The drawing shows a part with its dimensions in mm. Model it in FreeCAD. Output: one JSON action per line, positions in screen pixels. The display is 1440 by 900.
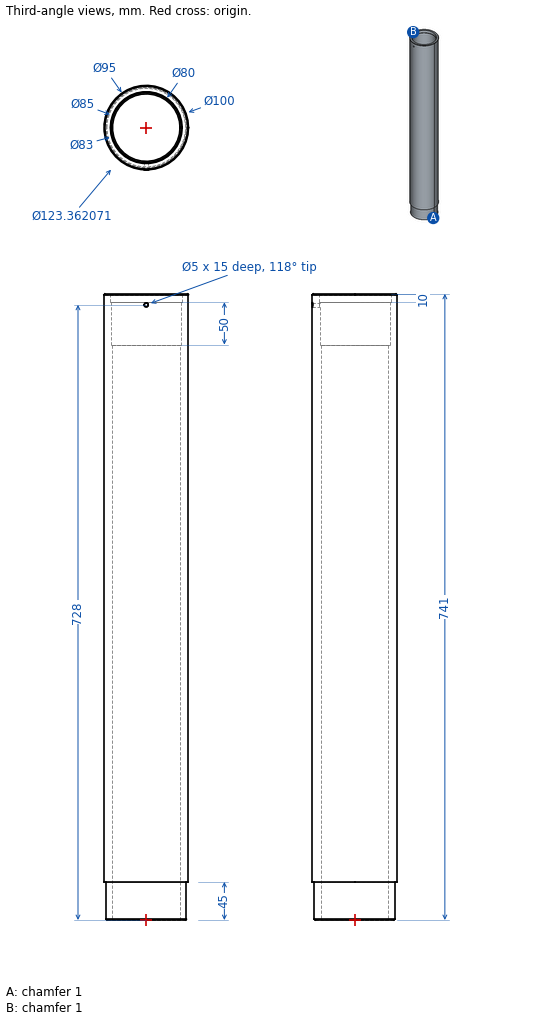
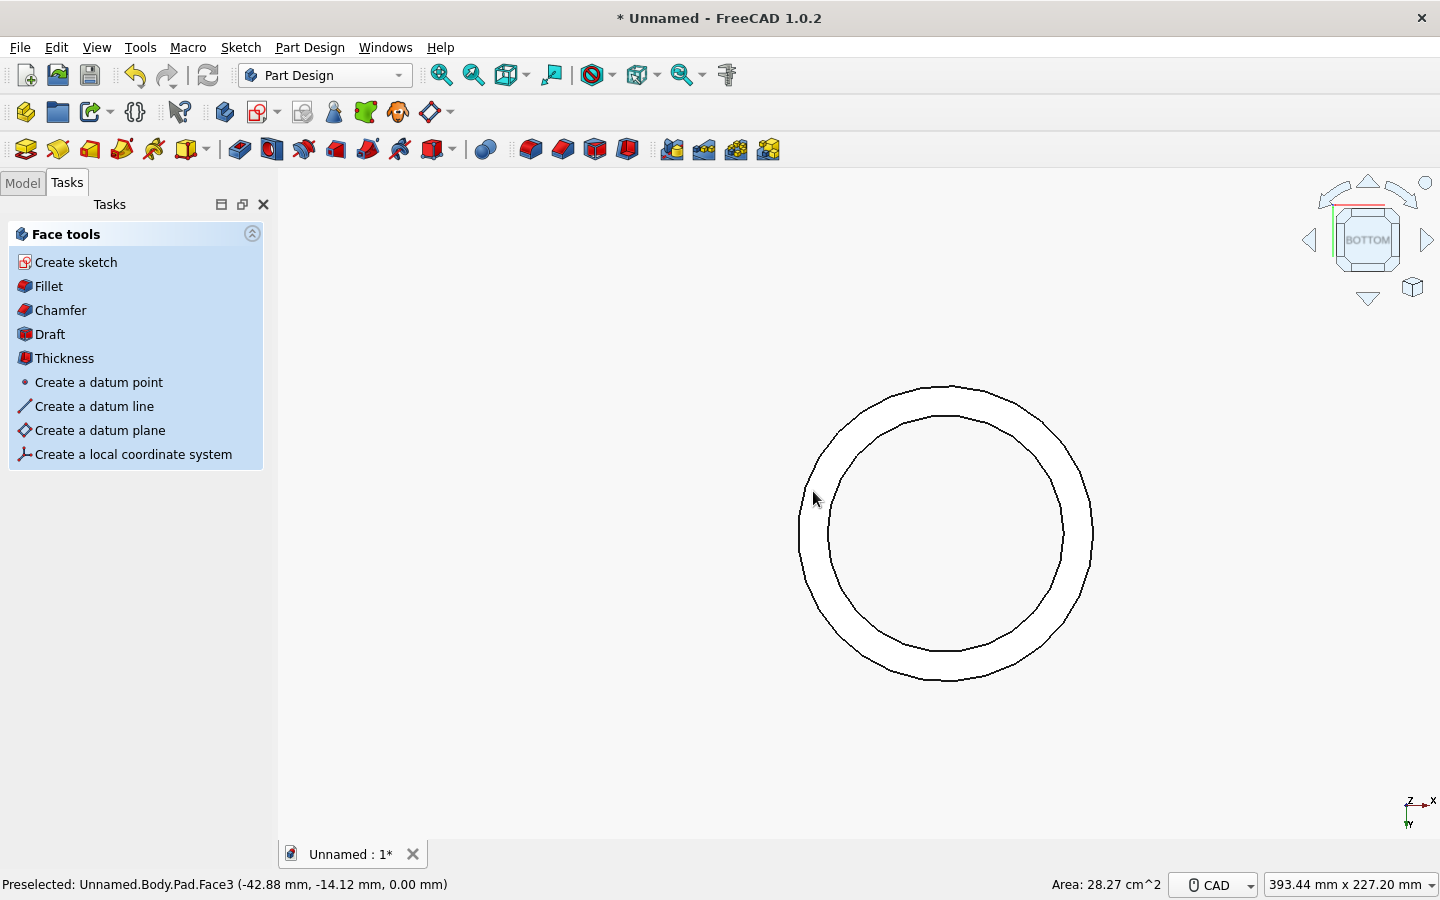
{"action": "left_click", "coordinate": [258, 112]}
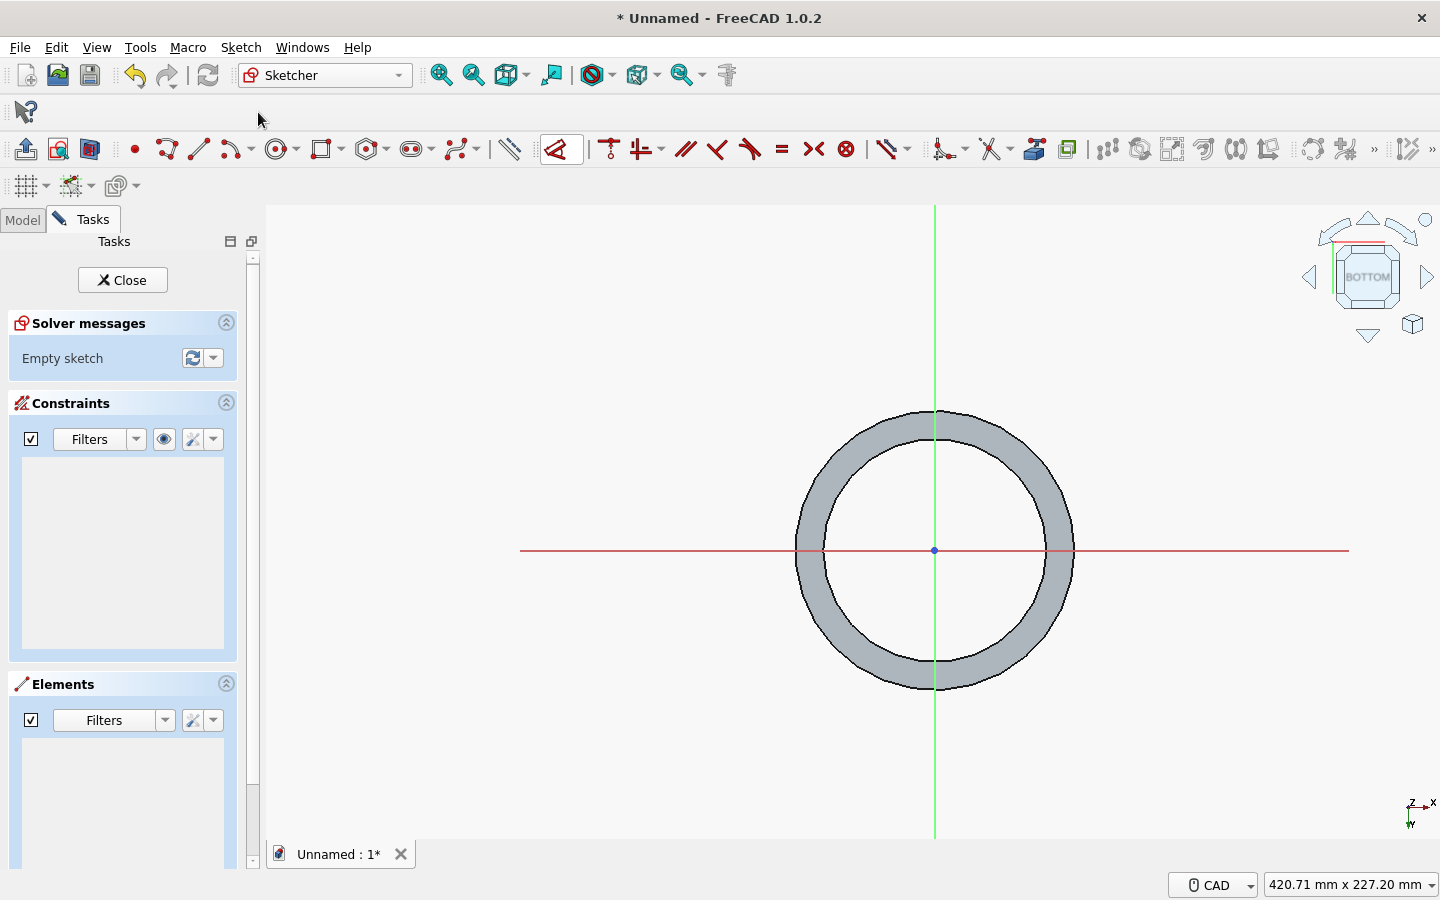
{"action": "left_click", "coordinate": [276, 150]}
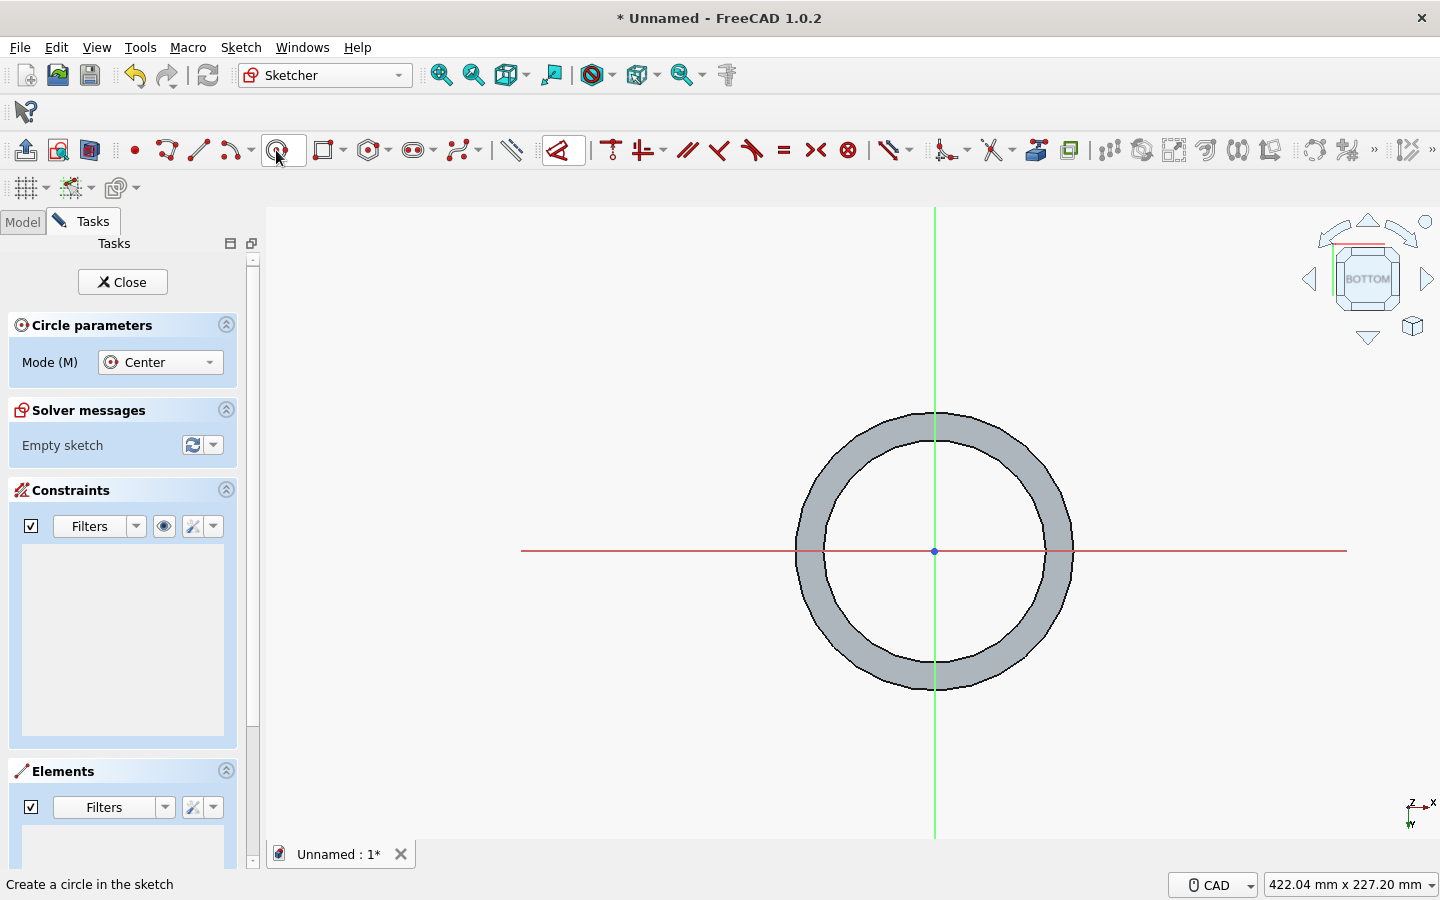
{"action": "left_click", "coordinate": [935, 551]}
{"action": "left_click", "coordinate": [1056, 430]}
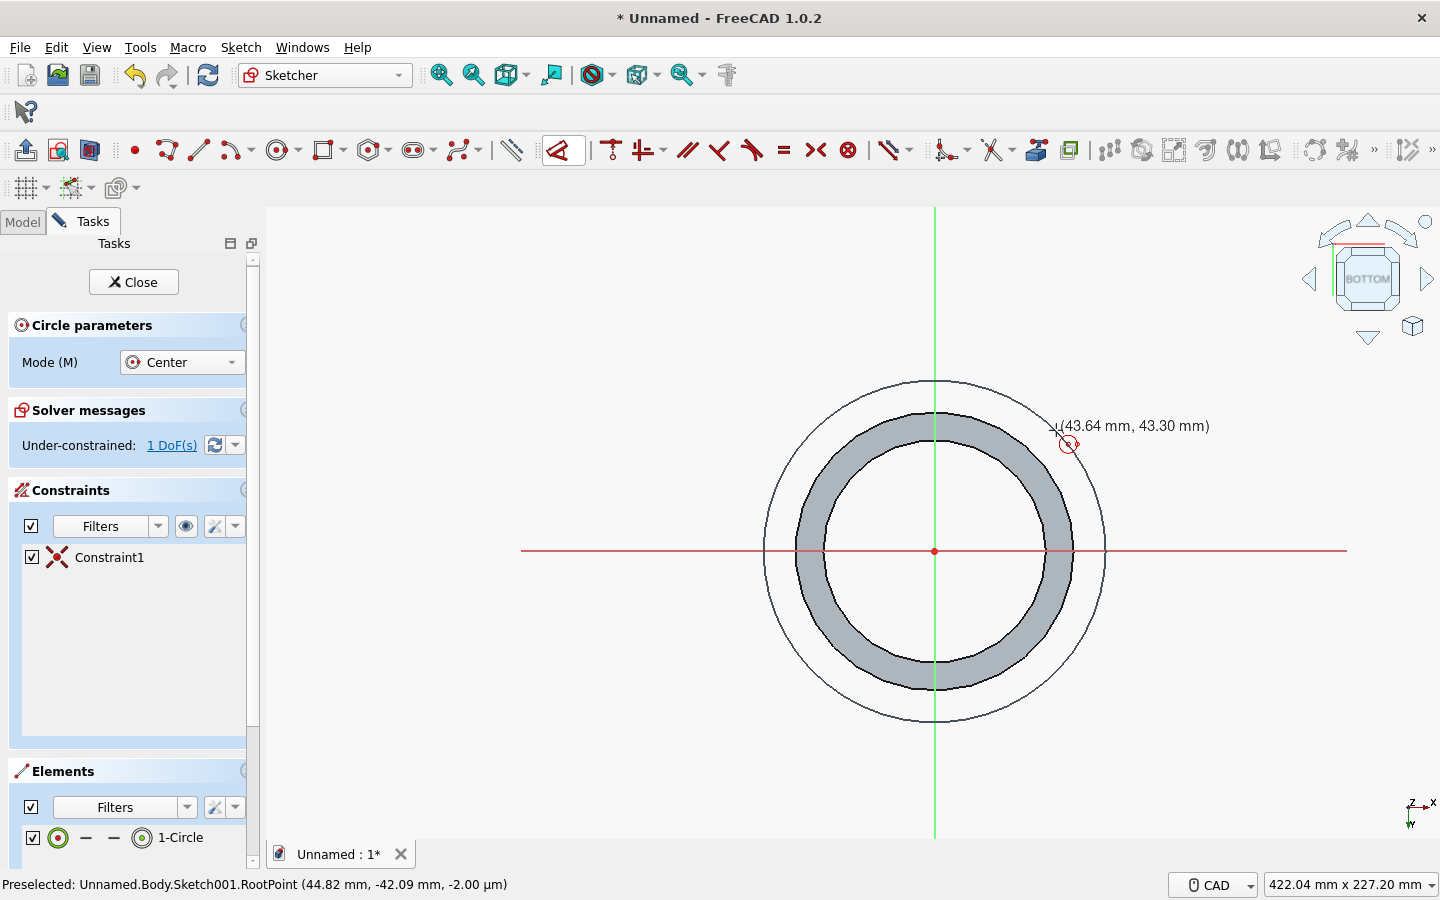
{"action": "left_click", "coordinate": [935, 551]}
{"action": "left_click", "coordinate": [1028, 458]}
{"action": "key", "text": "Escape"}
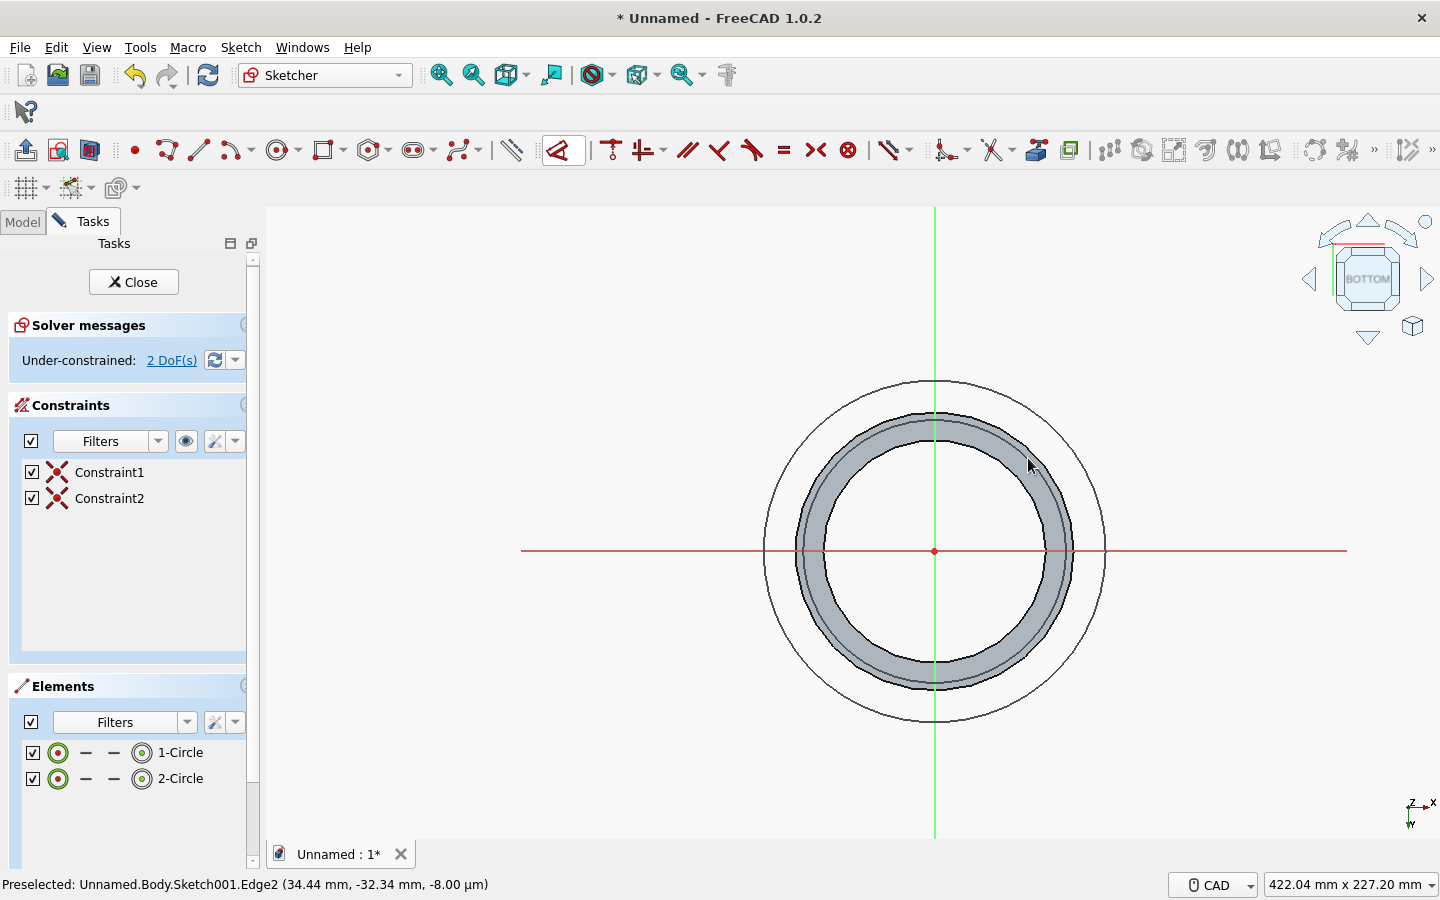
{"action": "left_click", "coordinate": [1055, 430]}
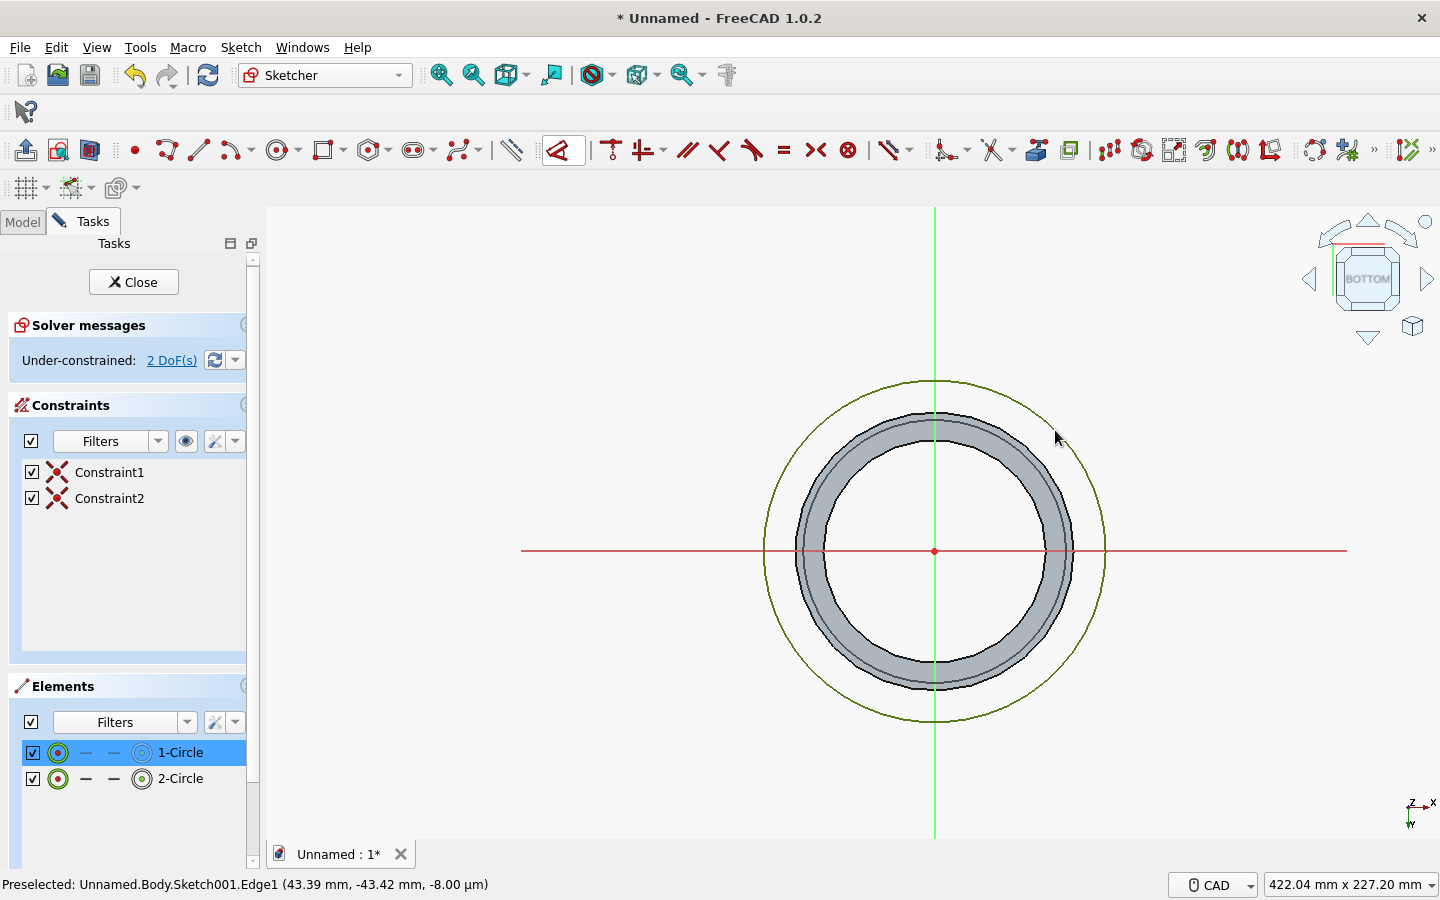
{"action": "key", "text": "k o"}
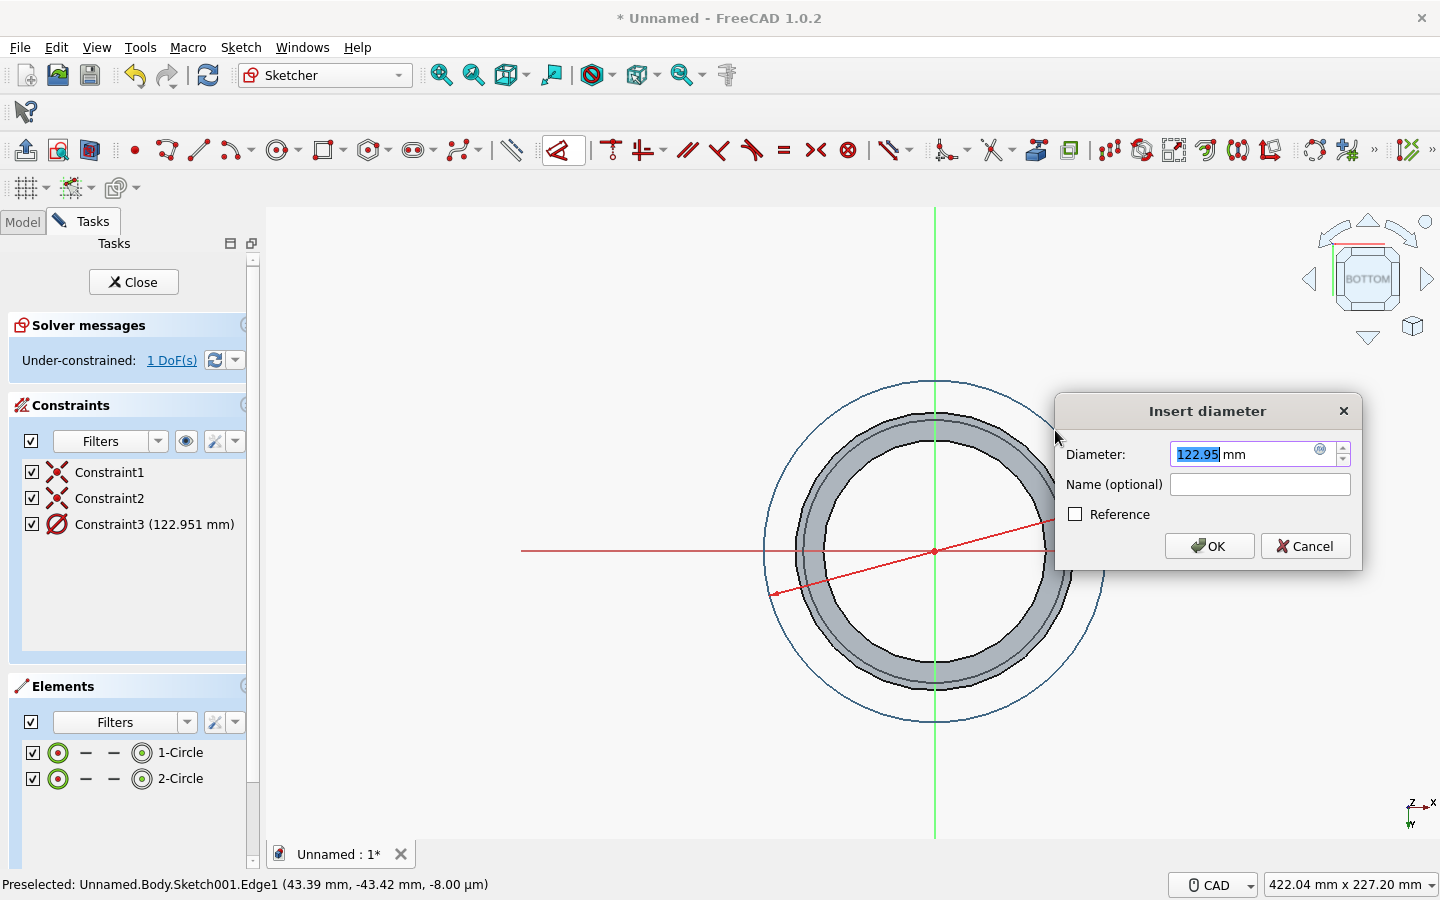
{"action": "type", "text": "123.362071"}
{"action": "key", "text": "Return"}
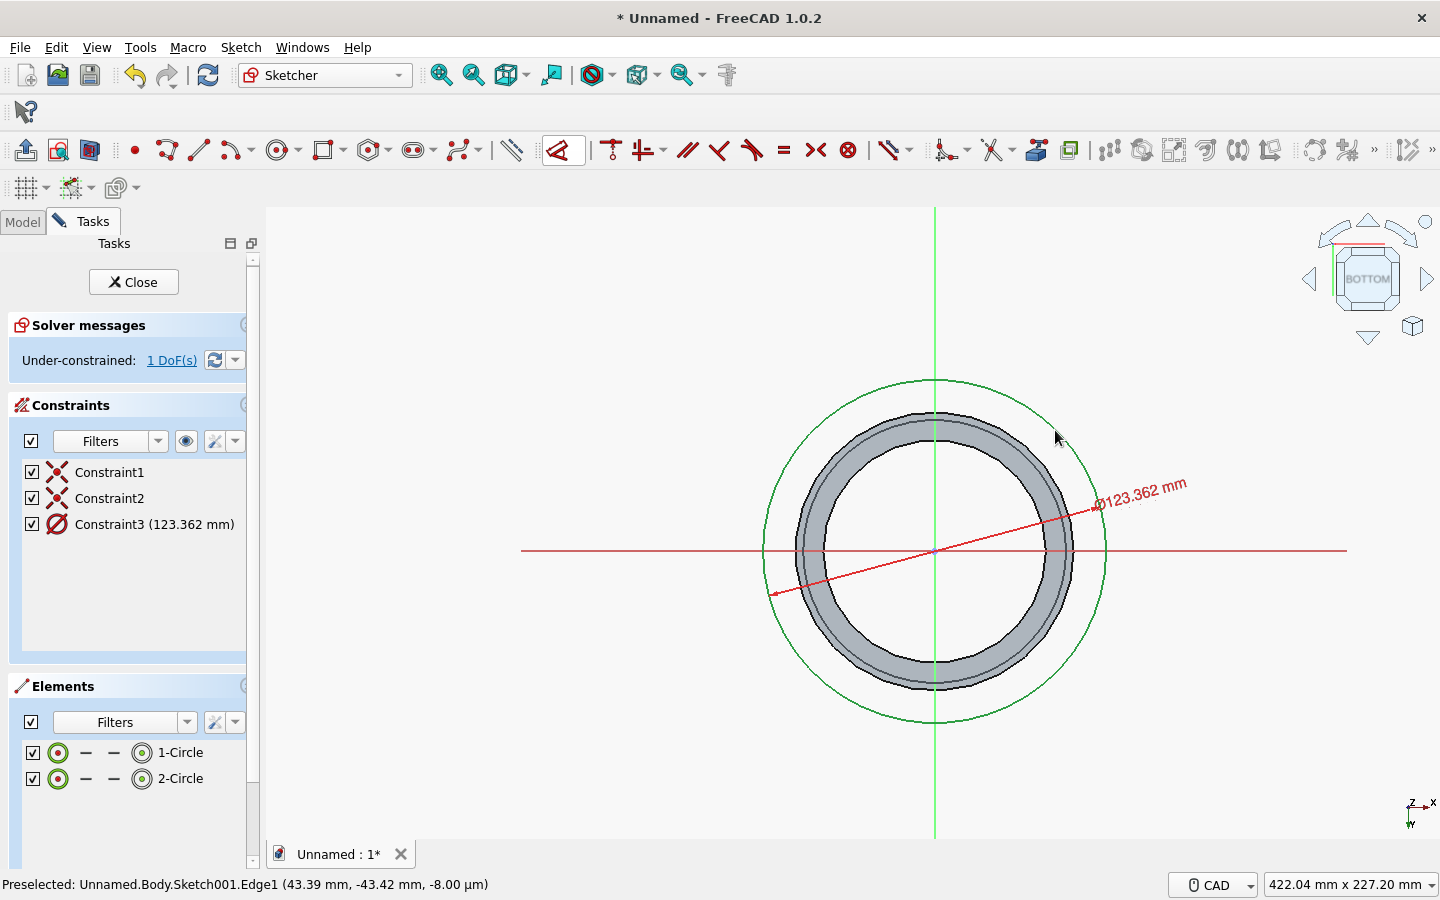
{"action": "left_click", "coordinate": [1027, 458]}